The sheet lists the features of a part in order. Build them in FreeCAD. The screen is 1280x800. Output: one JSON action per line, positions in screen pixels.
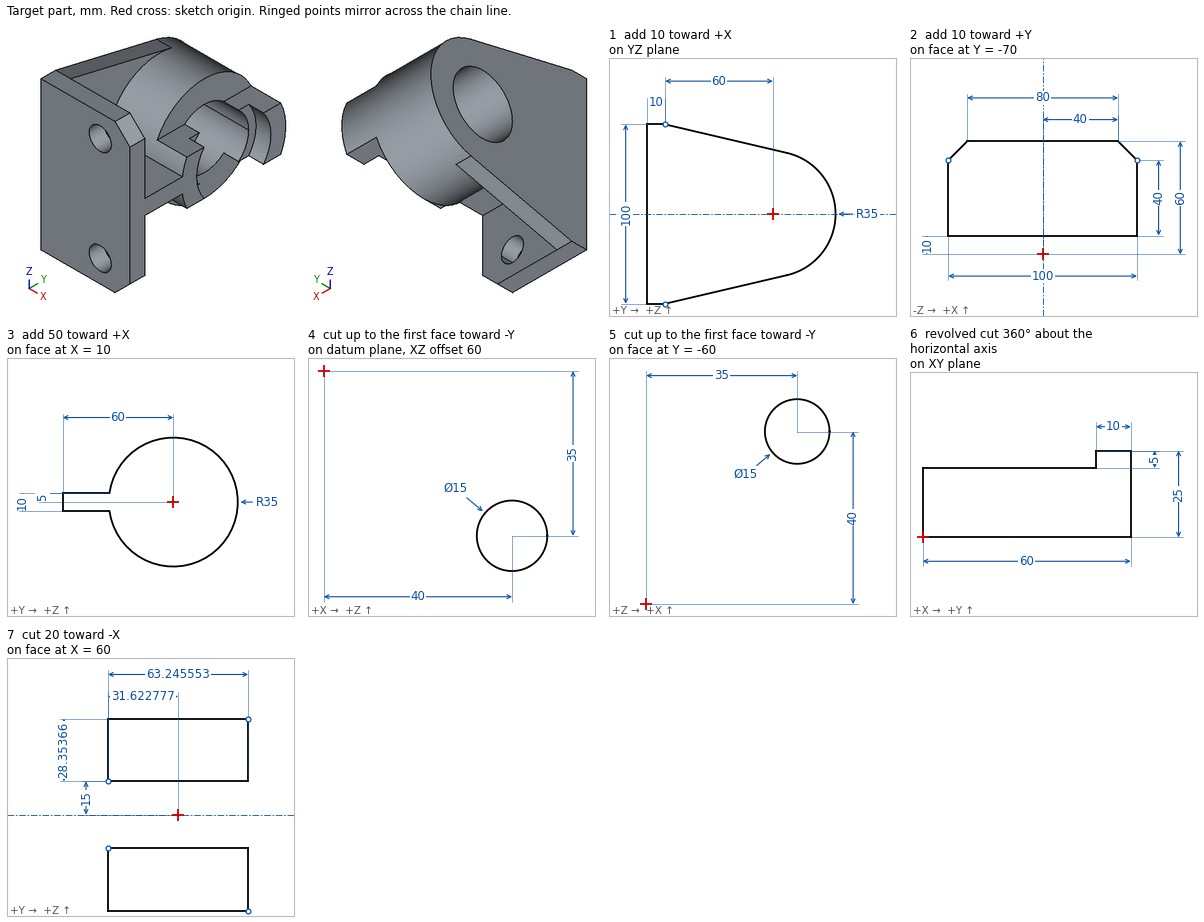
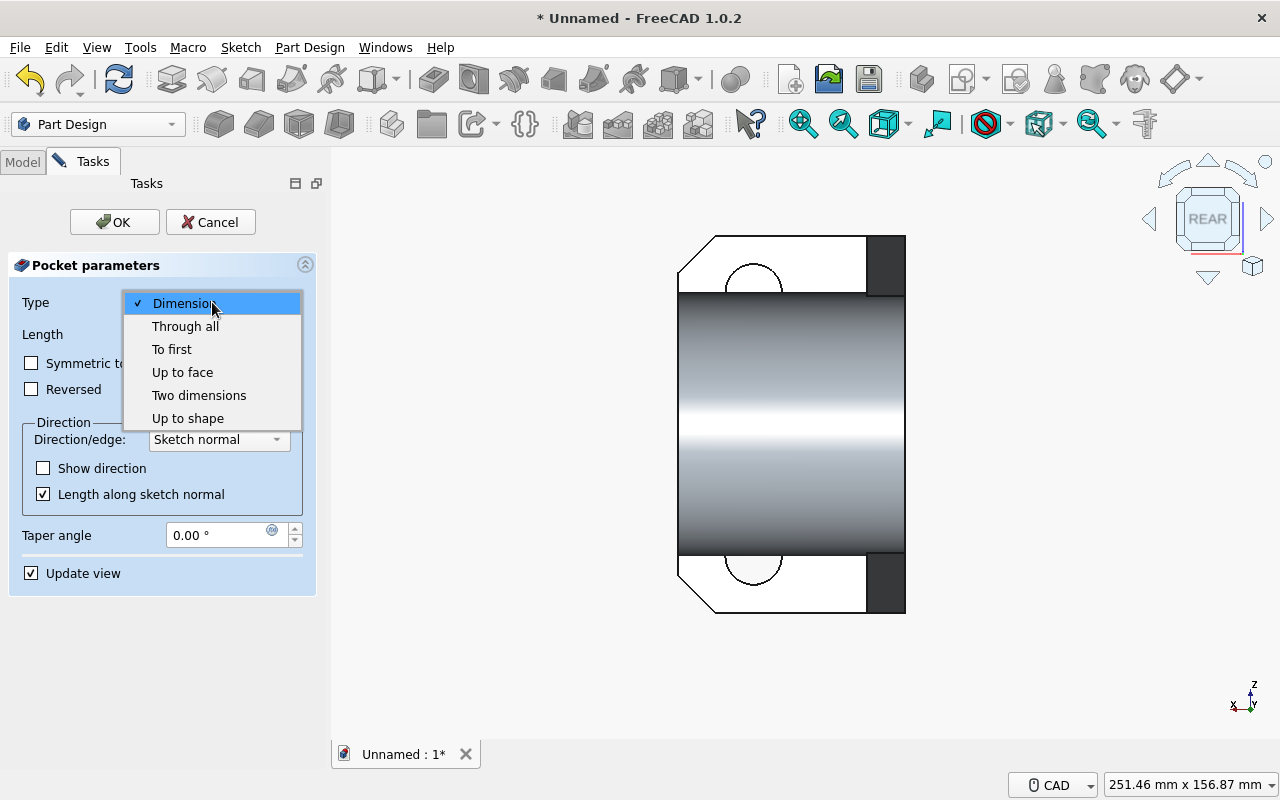
{"action": "left_click", "coordinate": [212, 350]}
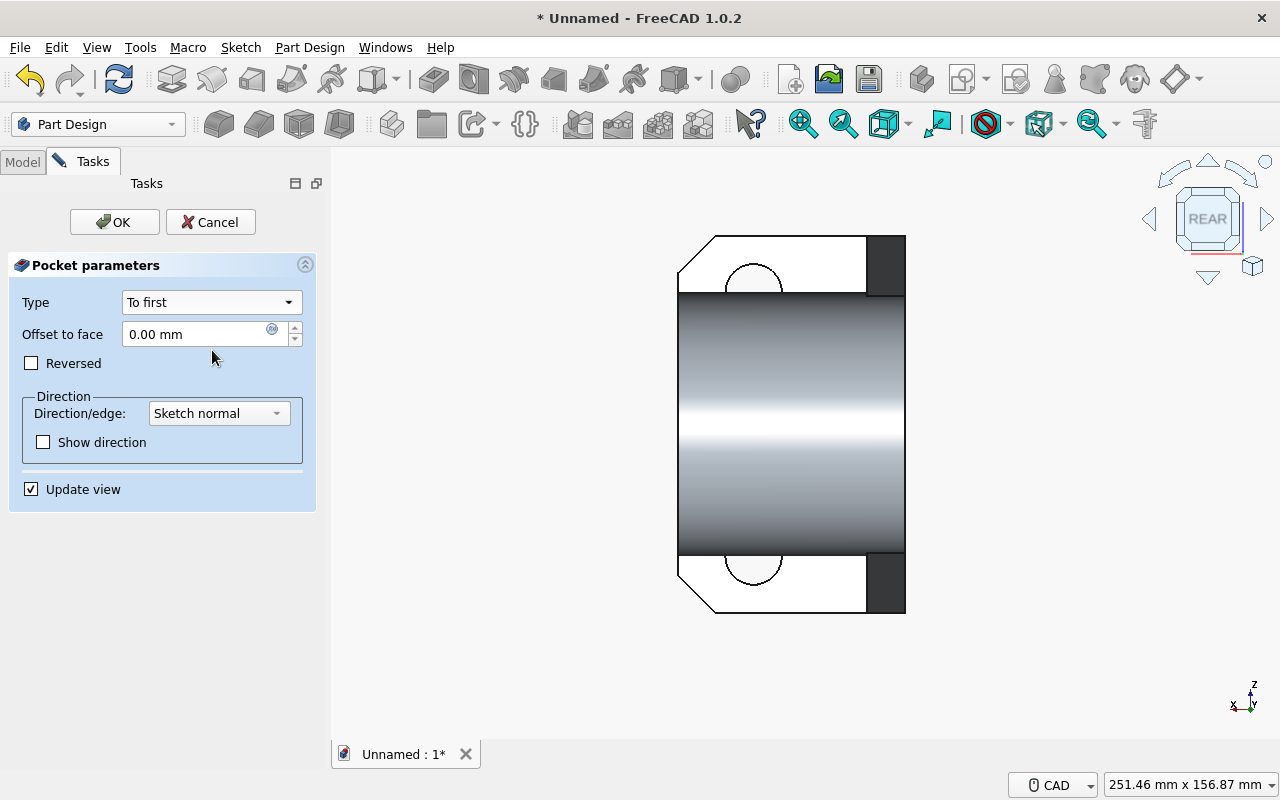
{"action": "left_click", "coordinate": [115, 222]}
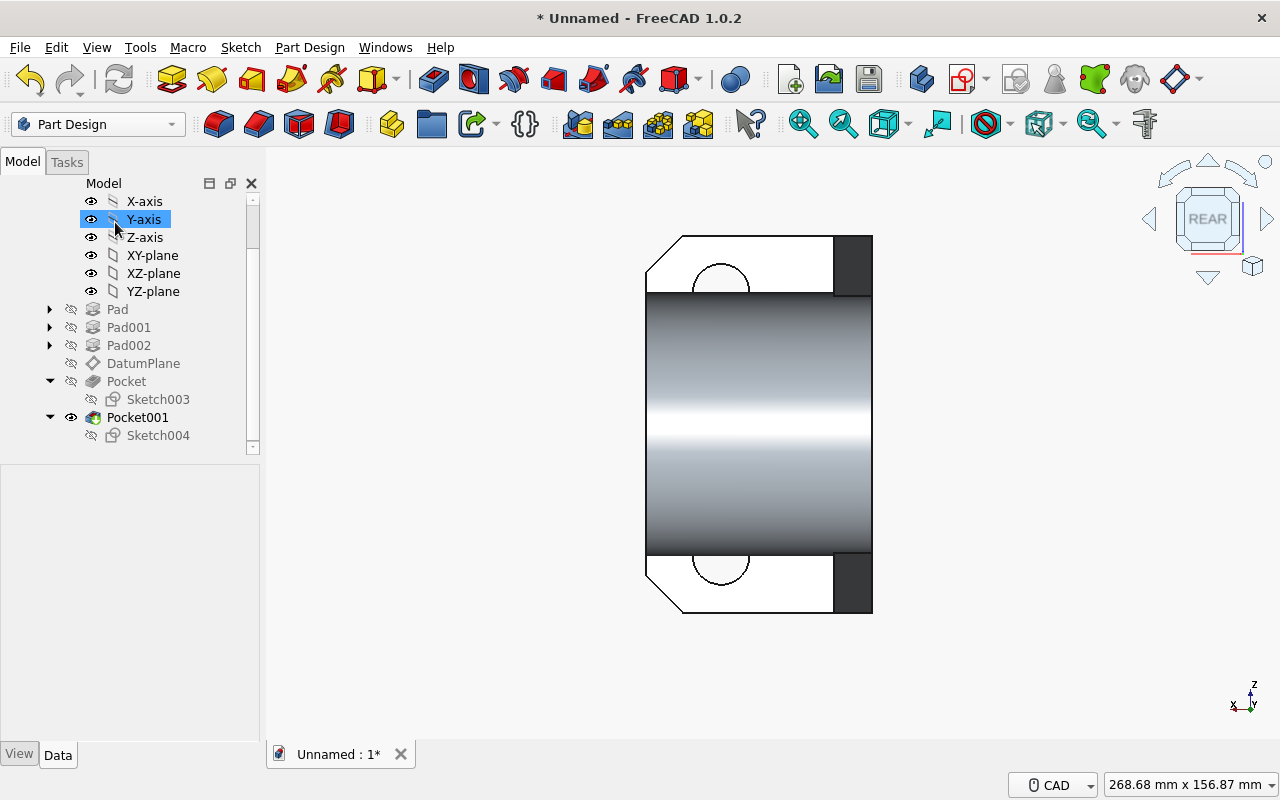
{"action": "left_click", "coordinate": [962, 80]}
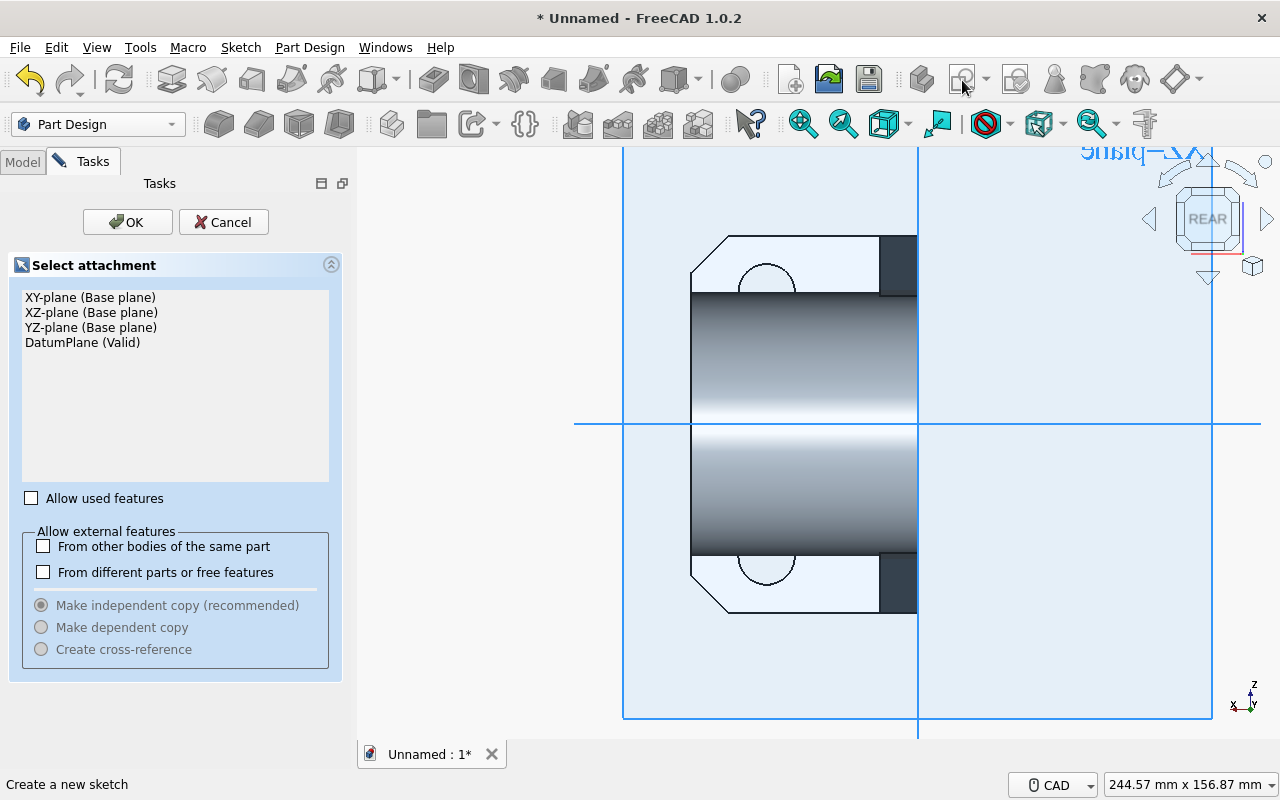
{"action": "left_click", "coordinate": [82, 298]}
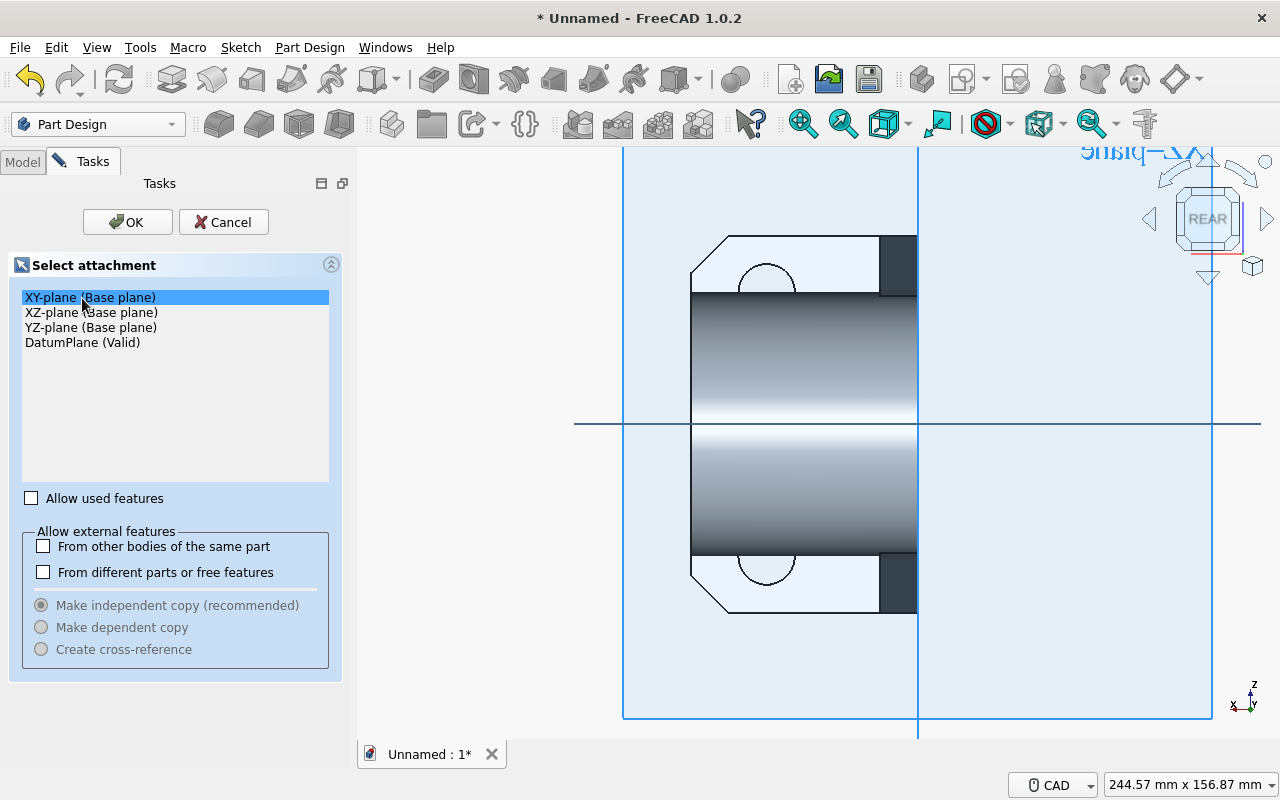
{"action": "left_click", "coordinate": [128, 222]}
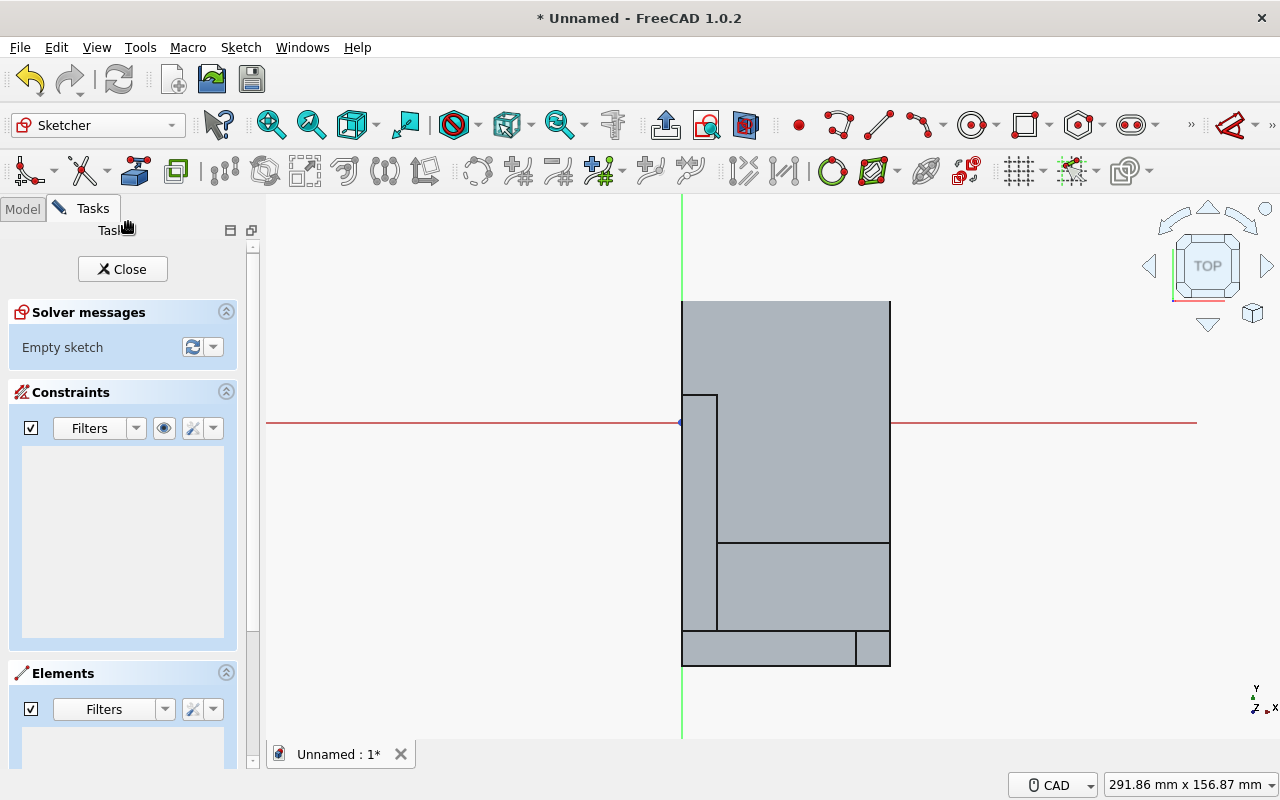
{"action": "left_click", "coordinate": [746, 126]}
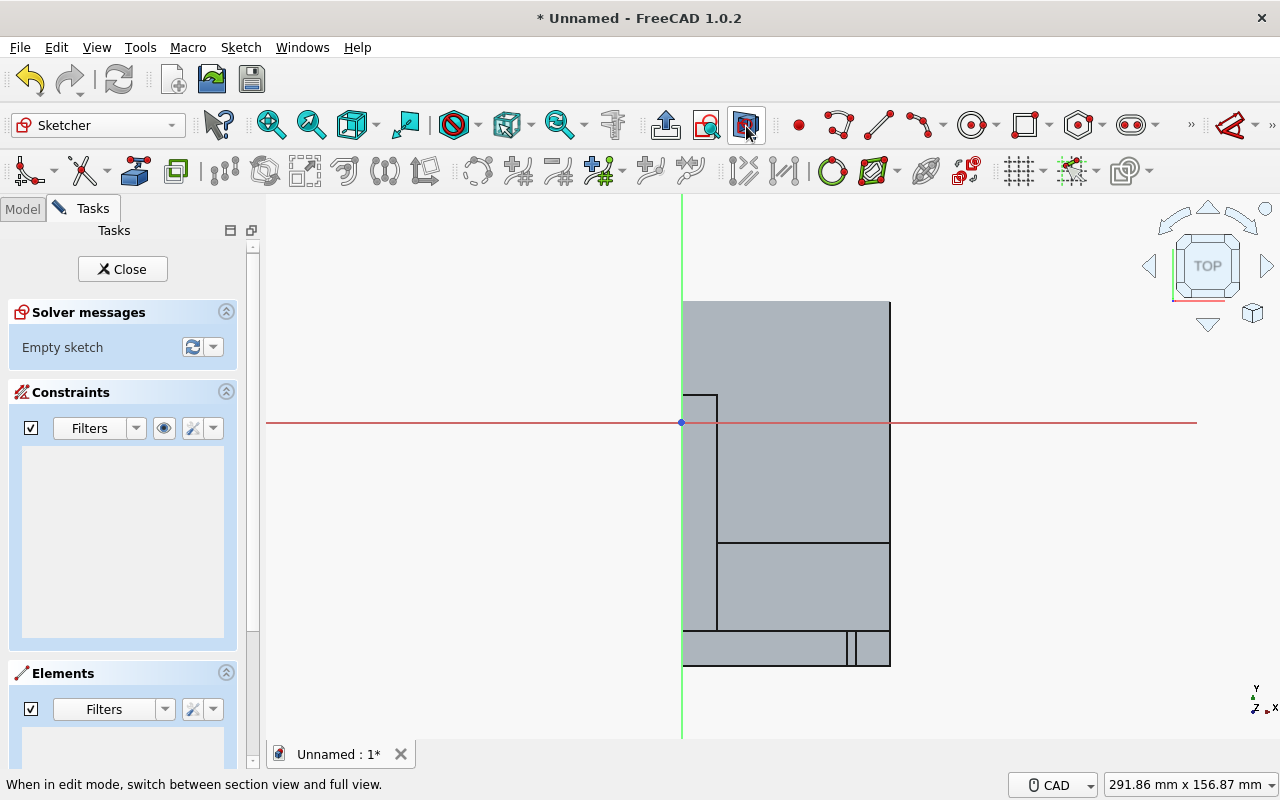
{"action": "scroll", "coordinate": [833, 329], "scroll_direction": "up", "scroll_amount": 5}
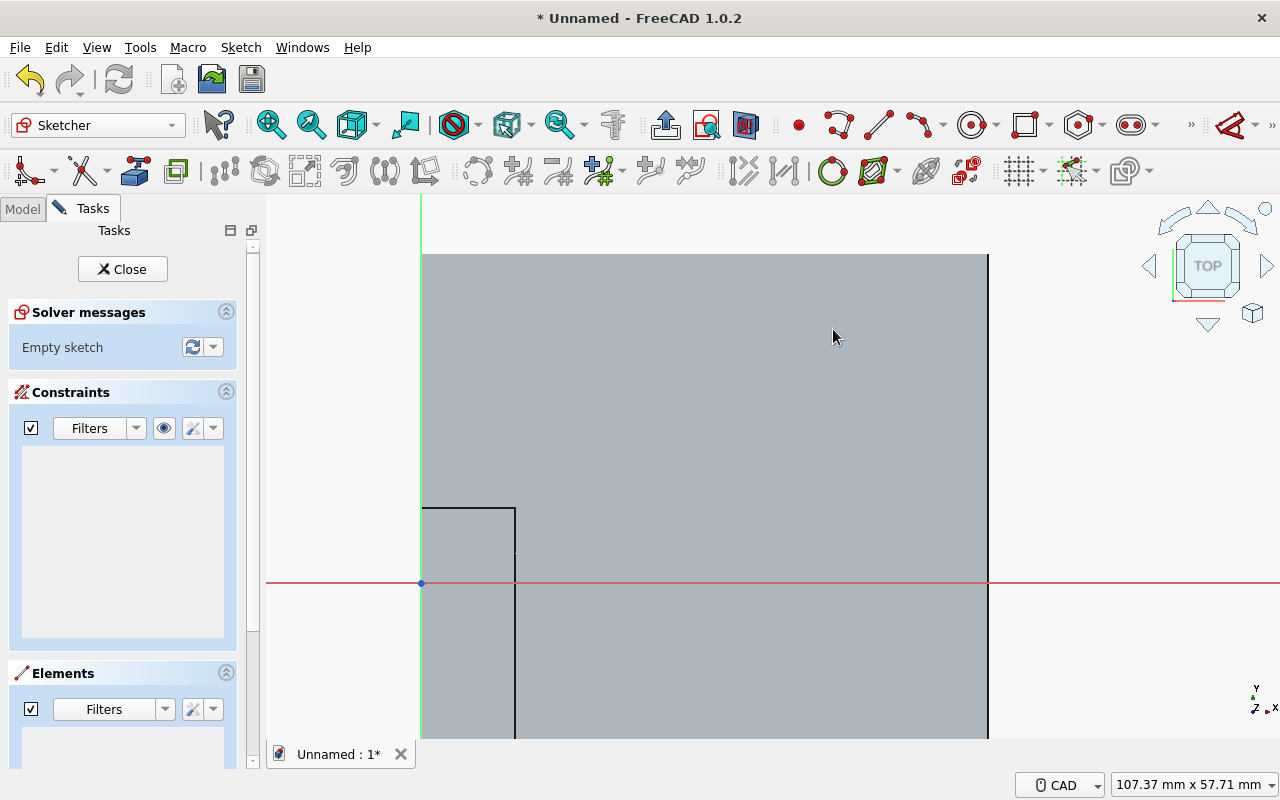
{"action": "left_click", "coordinate": [840, 126]}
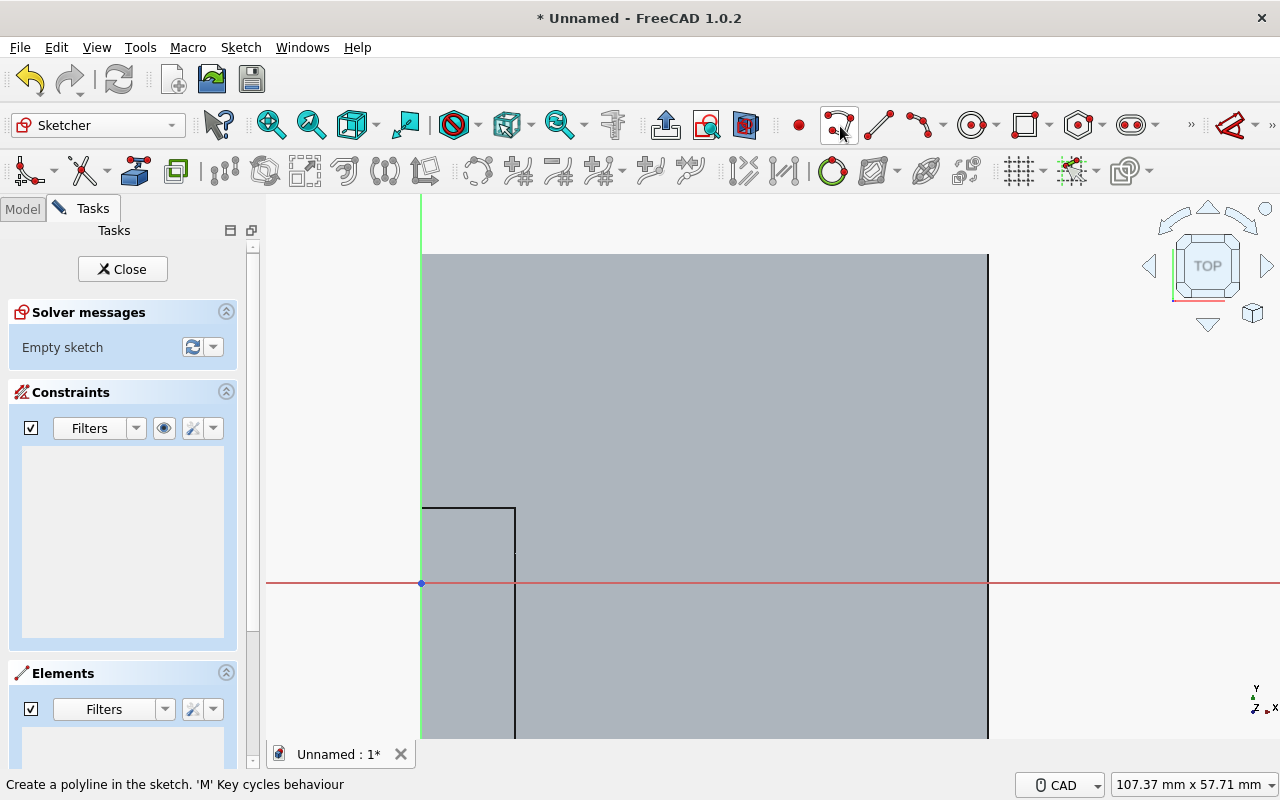
{"action": "left_click", "coordinate": [421, 583]}
{"action": "left_click", "coordinate": [988, 574]}
{"action": "left_click", "coordinate": [988, 347]}
{"action": "left_click", "coordinate": [893, 347]}
{"action": "left_click", "coordinate": [893, 395]}
{"action": "left_click", "coordinate": [430, 395]}
{"action": "left_click", "coordinate": [421, 583]}
{"action": "key", "text": "Escape"}
{"action": "key", "text": "Escape"}